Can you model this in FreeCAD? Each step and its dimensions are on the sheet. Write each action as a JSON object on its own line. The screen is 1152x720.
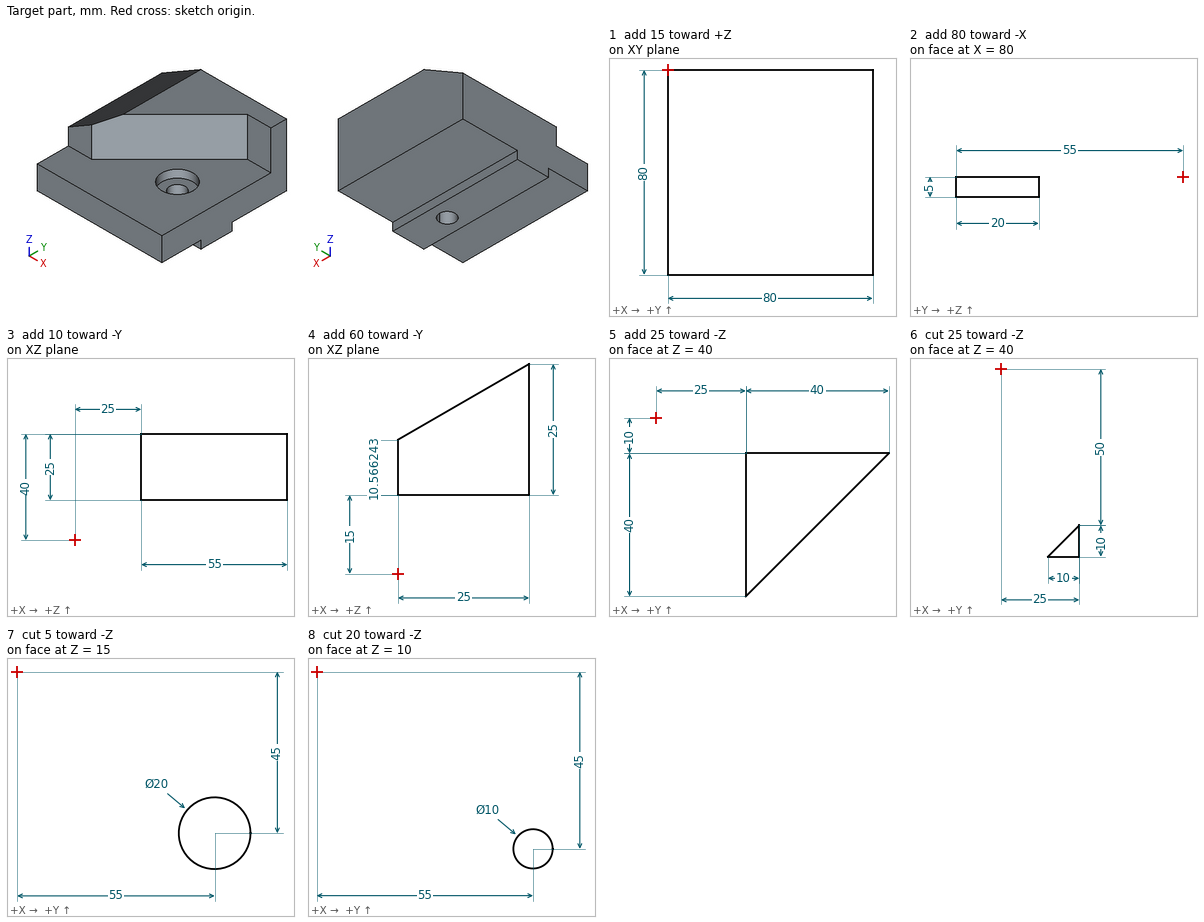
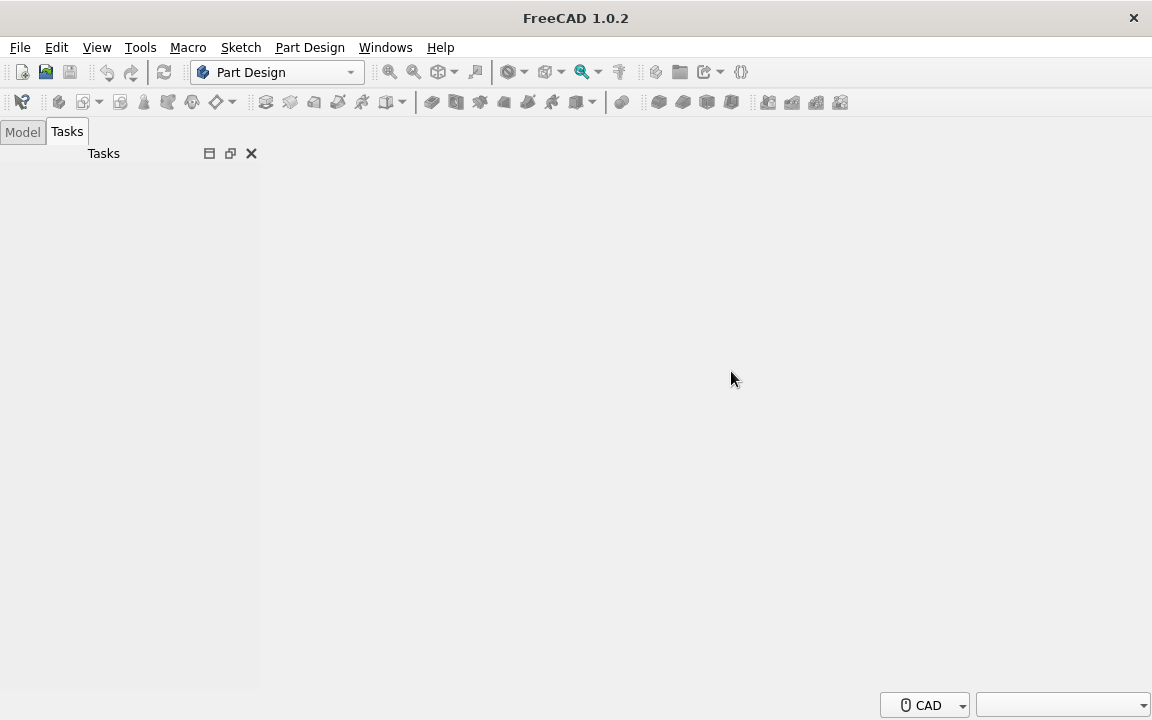
{"action": "left_click", "coordinate": [22, 72]}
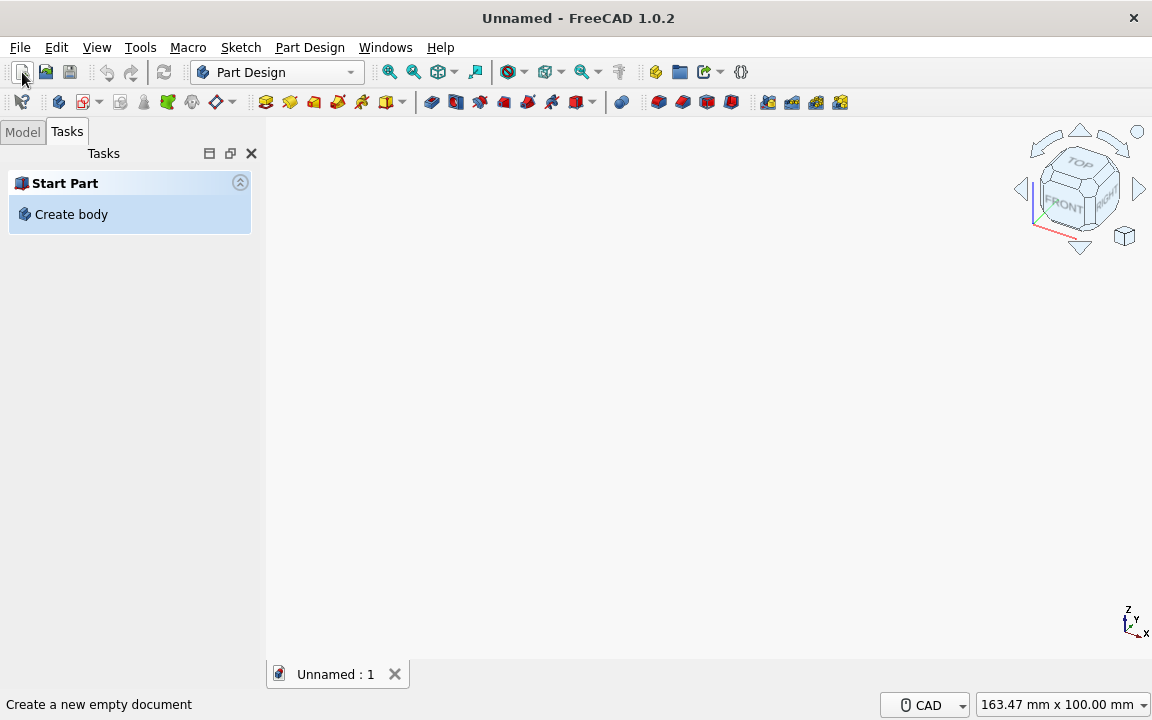
{"action": "left_click", "coordinate": [84, 102]}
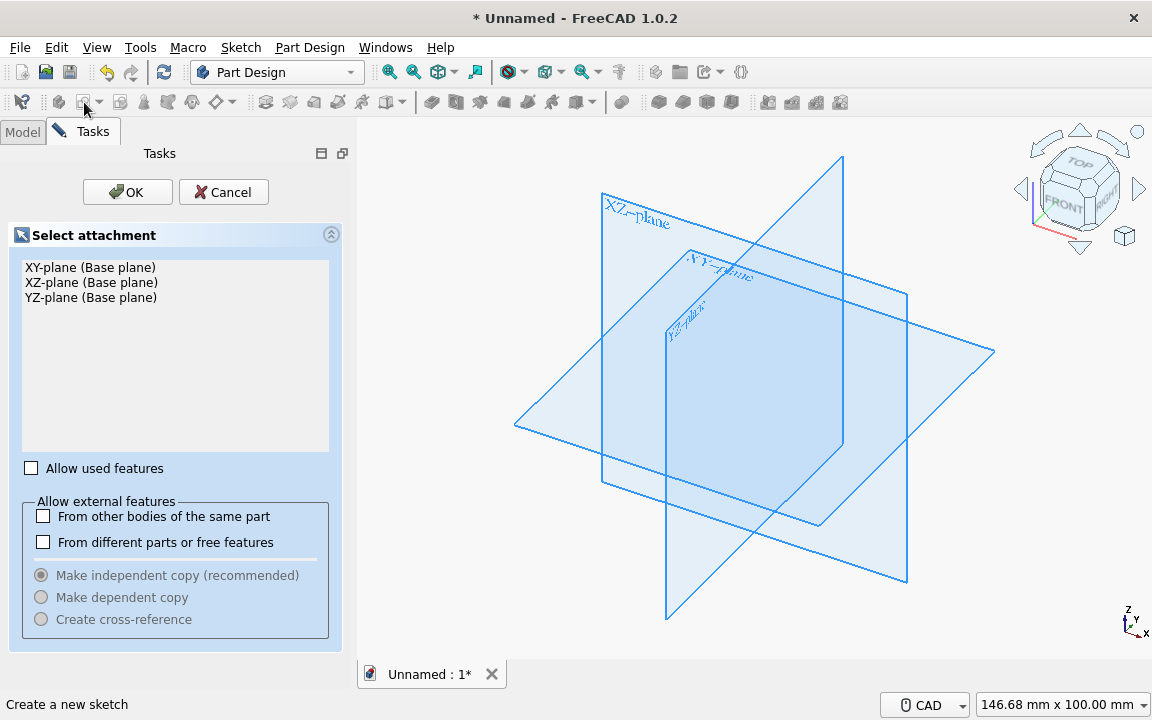
{"action": "left_click", "coordinate": [82, 268]}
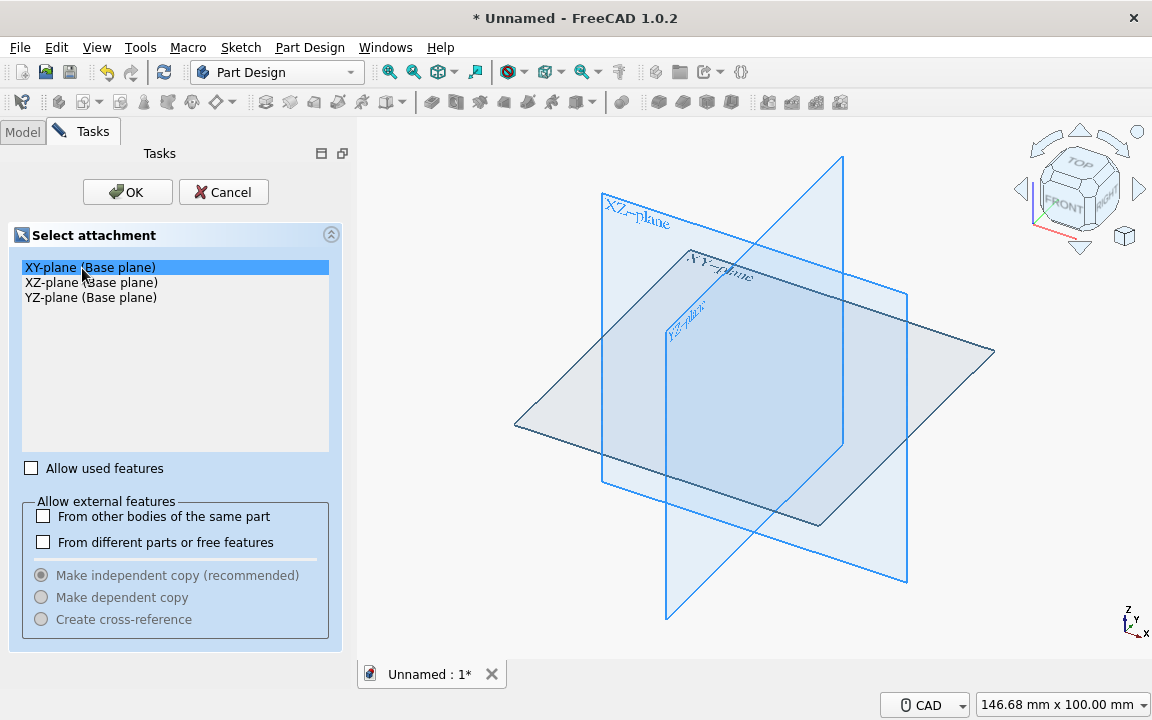
{"action": "left_click", "coordinate": [128, 192]}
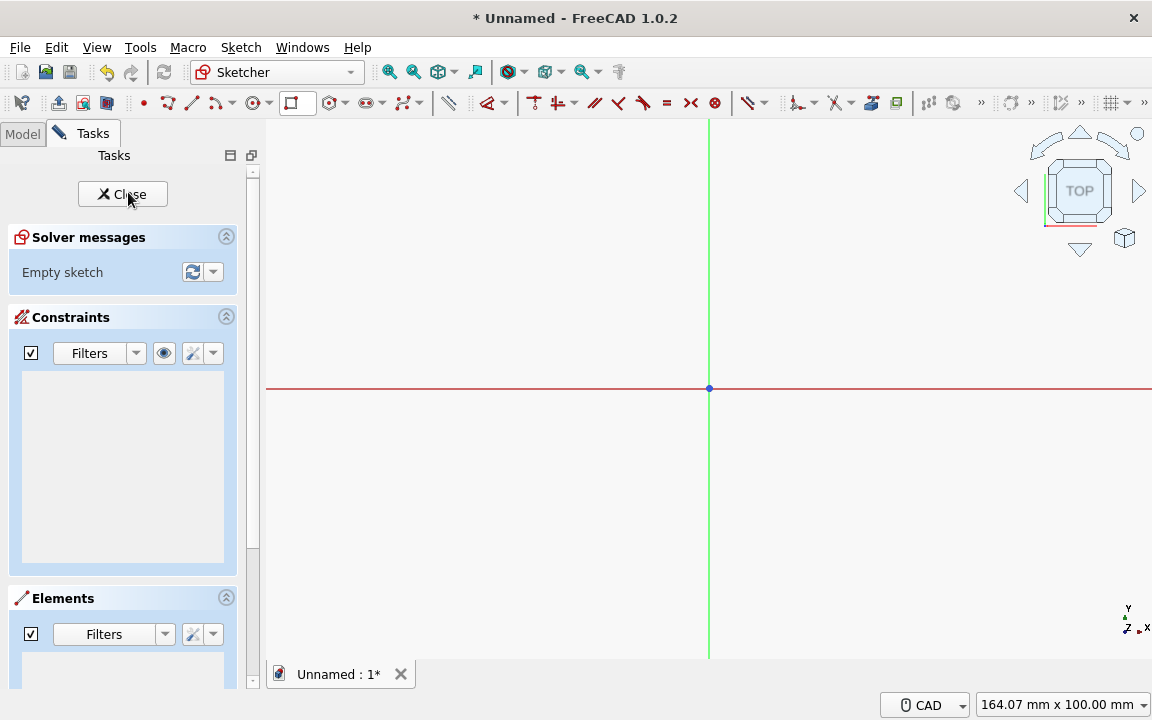
{"action": "scroll", "coordinate": [294, 147], "scroll_direction": "down", "scroll_amount": 2}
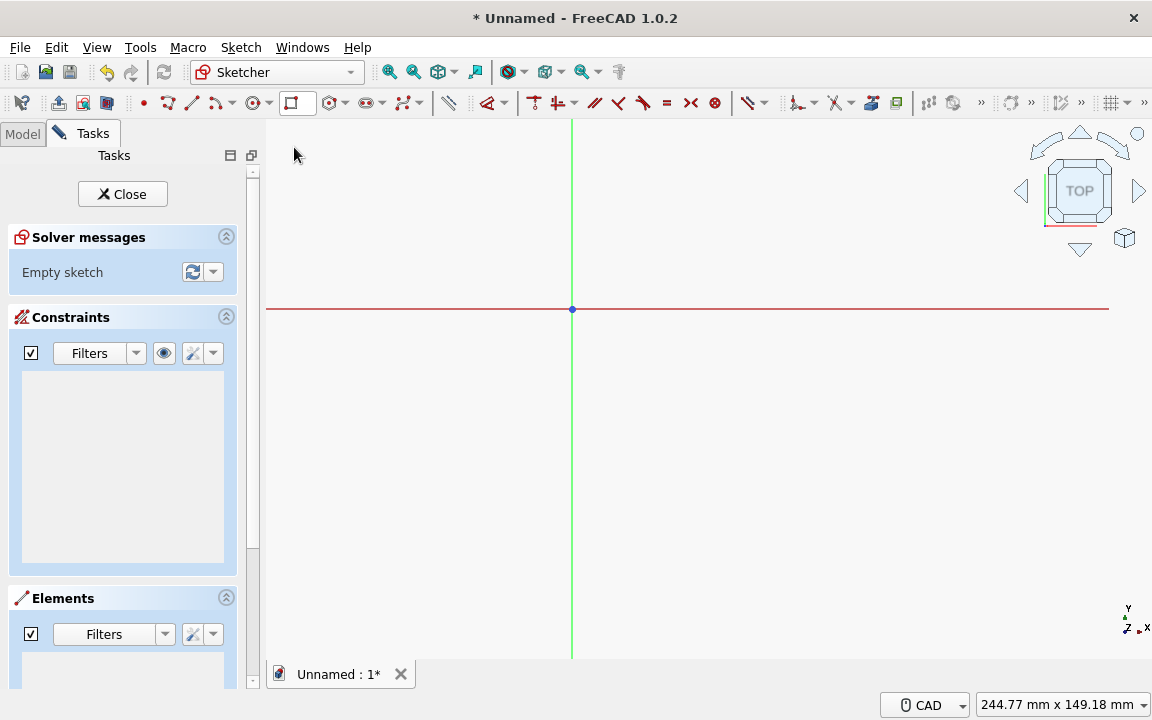
{"action": "left_click", "coordinate": [292, 104]}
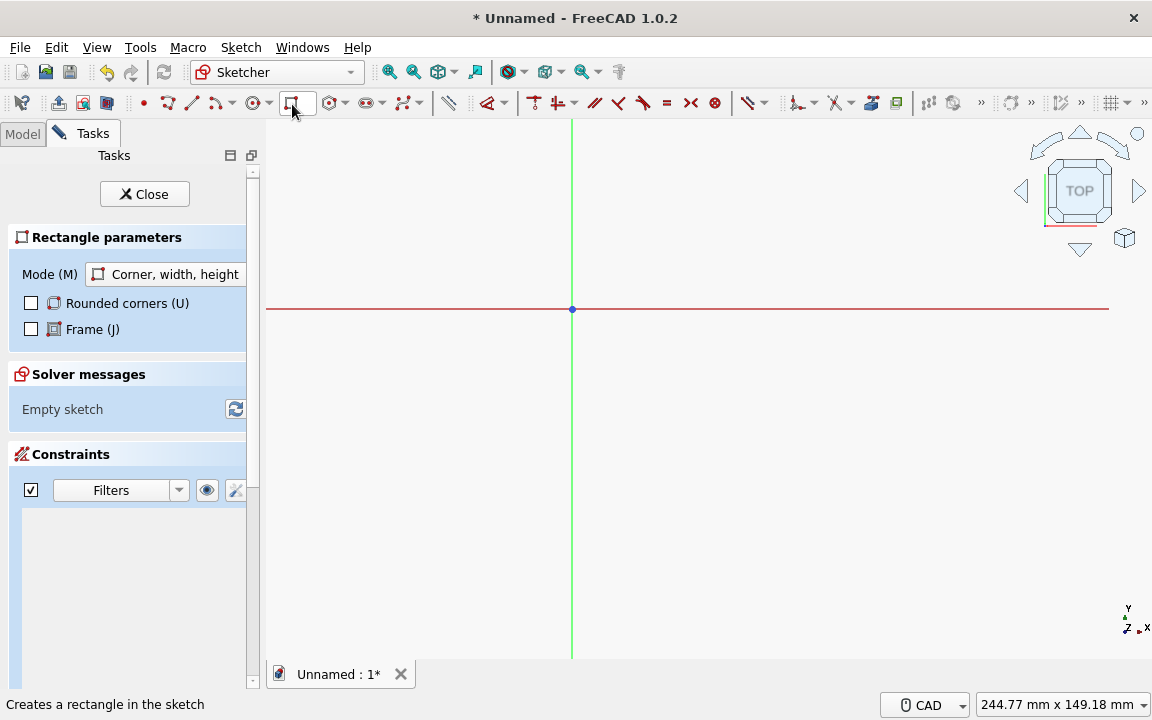
{"action": "left_click", "coordinate": [572, 309]}
{"action": "left_click", "coordinate": [862, 599]}
{"action": "key", "text": "Escape"}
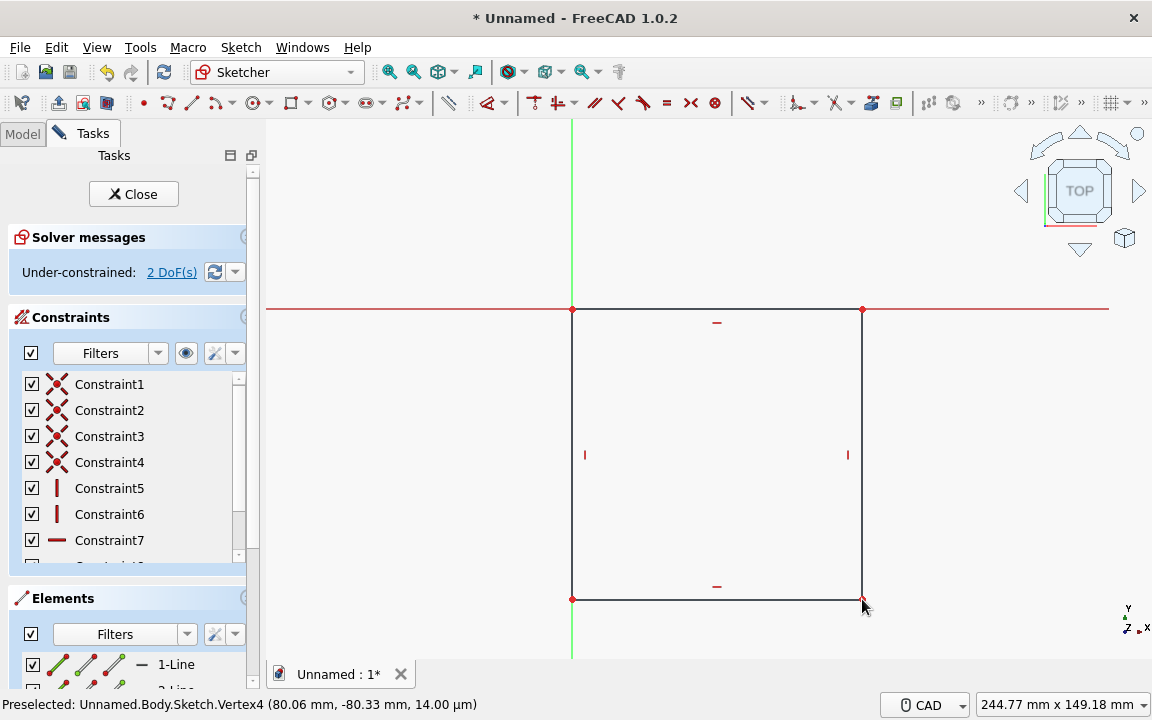
{"action": "left_click", "coordinate": [488, 104]}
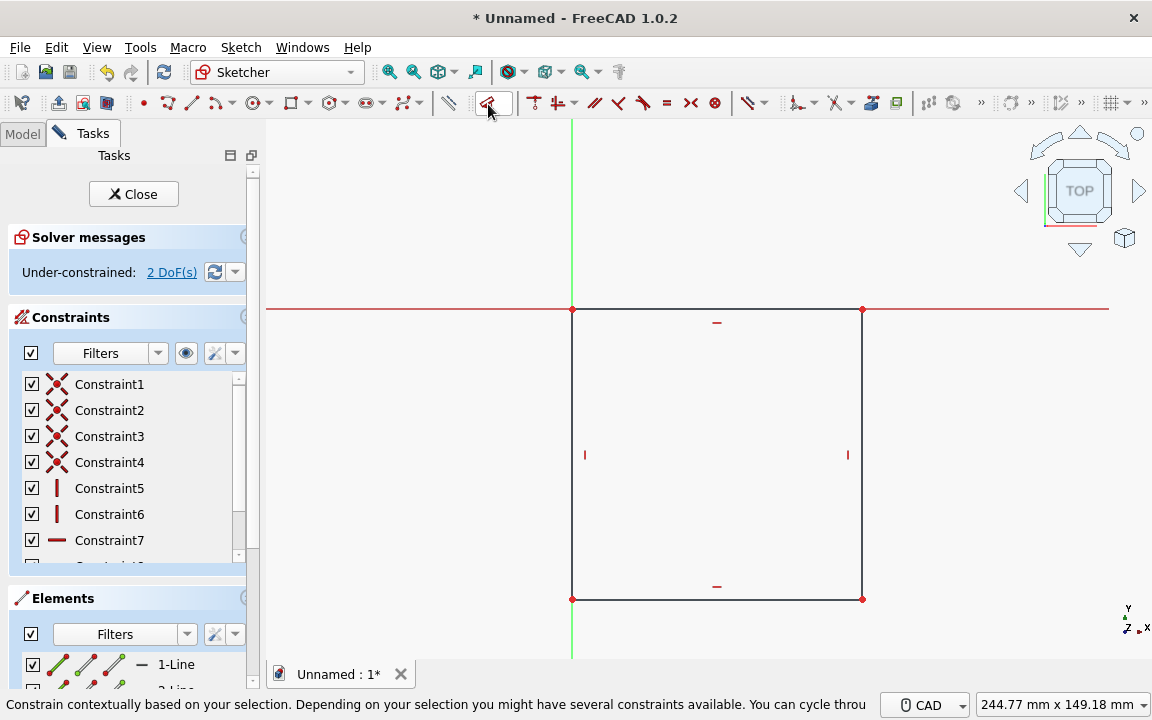
{"action": "left_click", "coordinate": [572, 396]}
{"action": "left_click", "coordinate": [538, 455]}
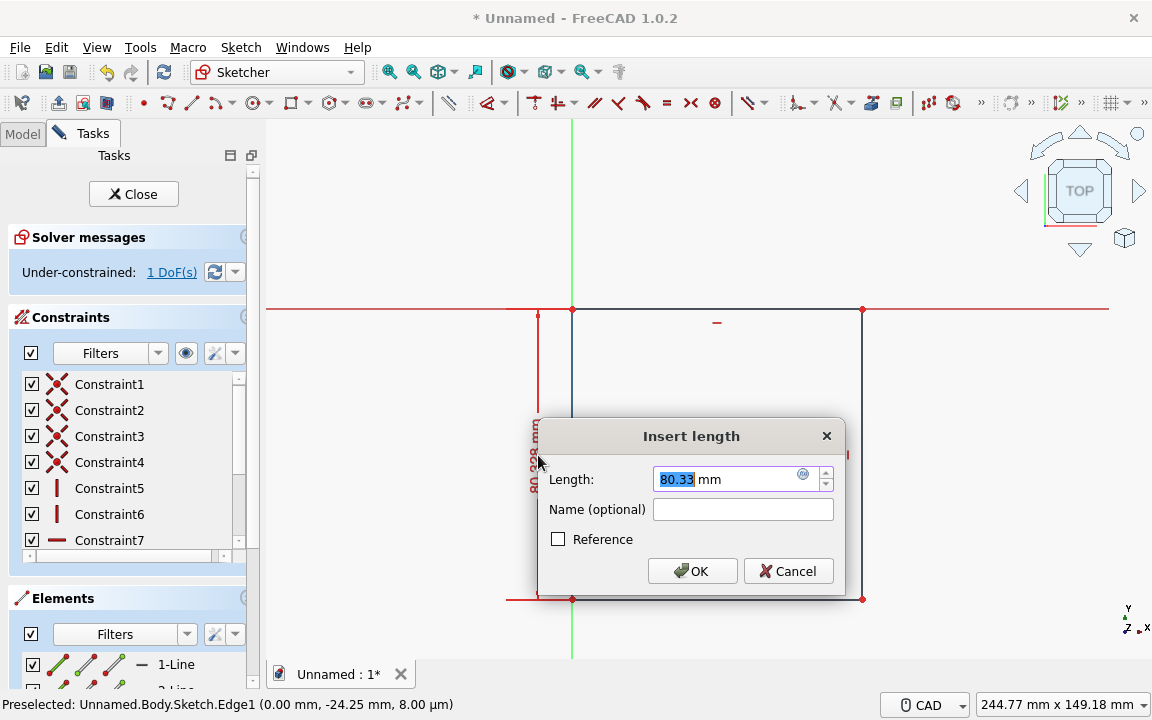
{"action": "type", "text": "80"}
{"action": "key", "text": "Return"}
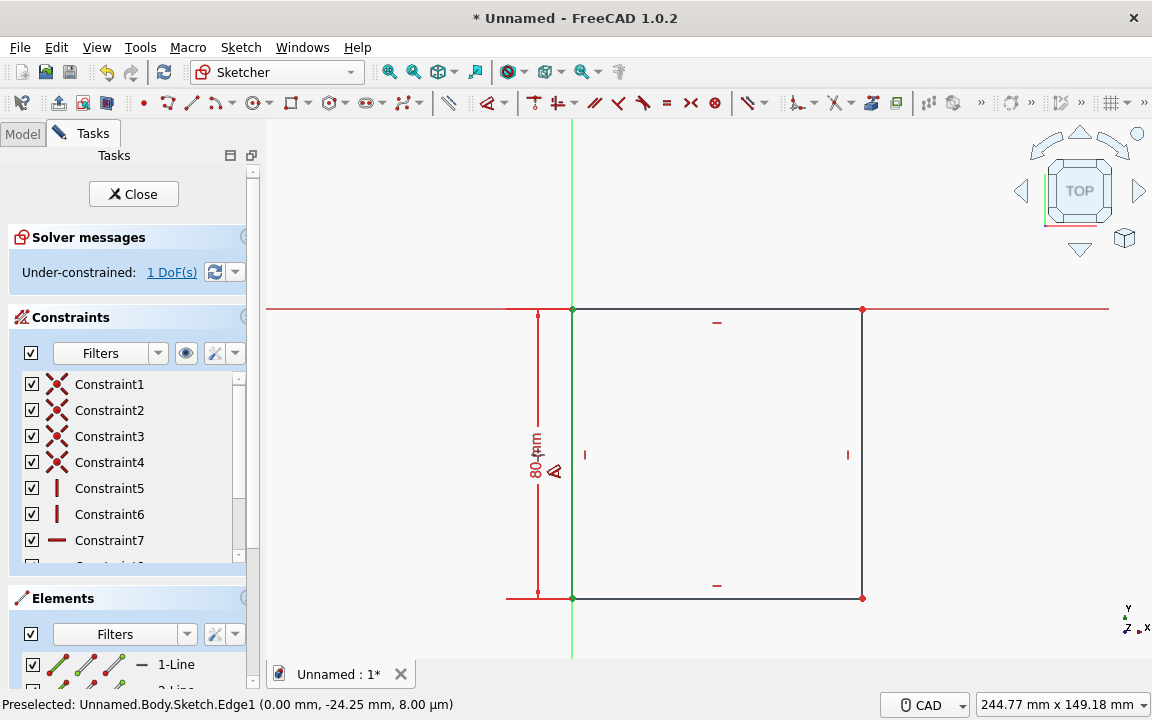
{"action": "left_click", "coordinate": [659, 599]}
{"action": "left_click", "coordinate": [717, 565]}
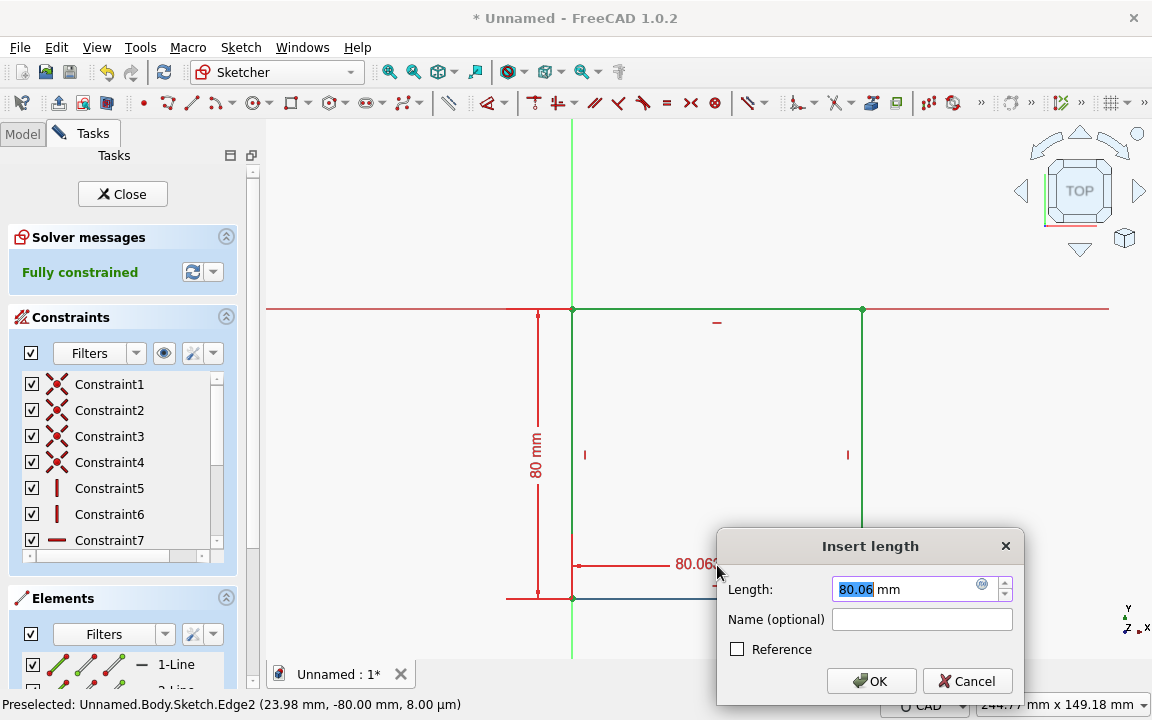
{"action": "type", "text": "80"}
{"action": "key", "text": "Return"}
{"action": "key", "text": "Escape"}